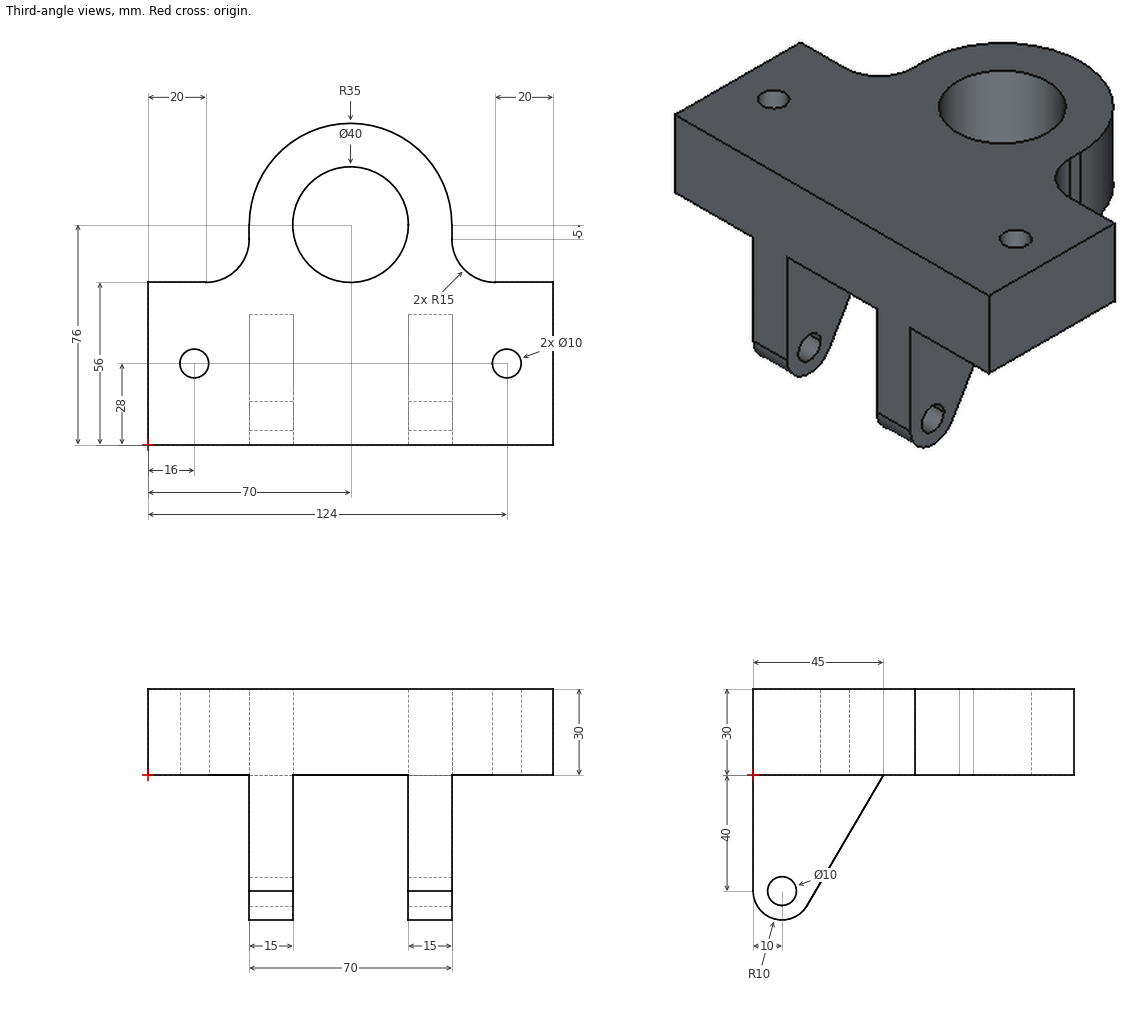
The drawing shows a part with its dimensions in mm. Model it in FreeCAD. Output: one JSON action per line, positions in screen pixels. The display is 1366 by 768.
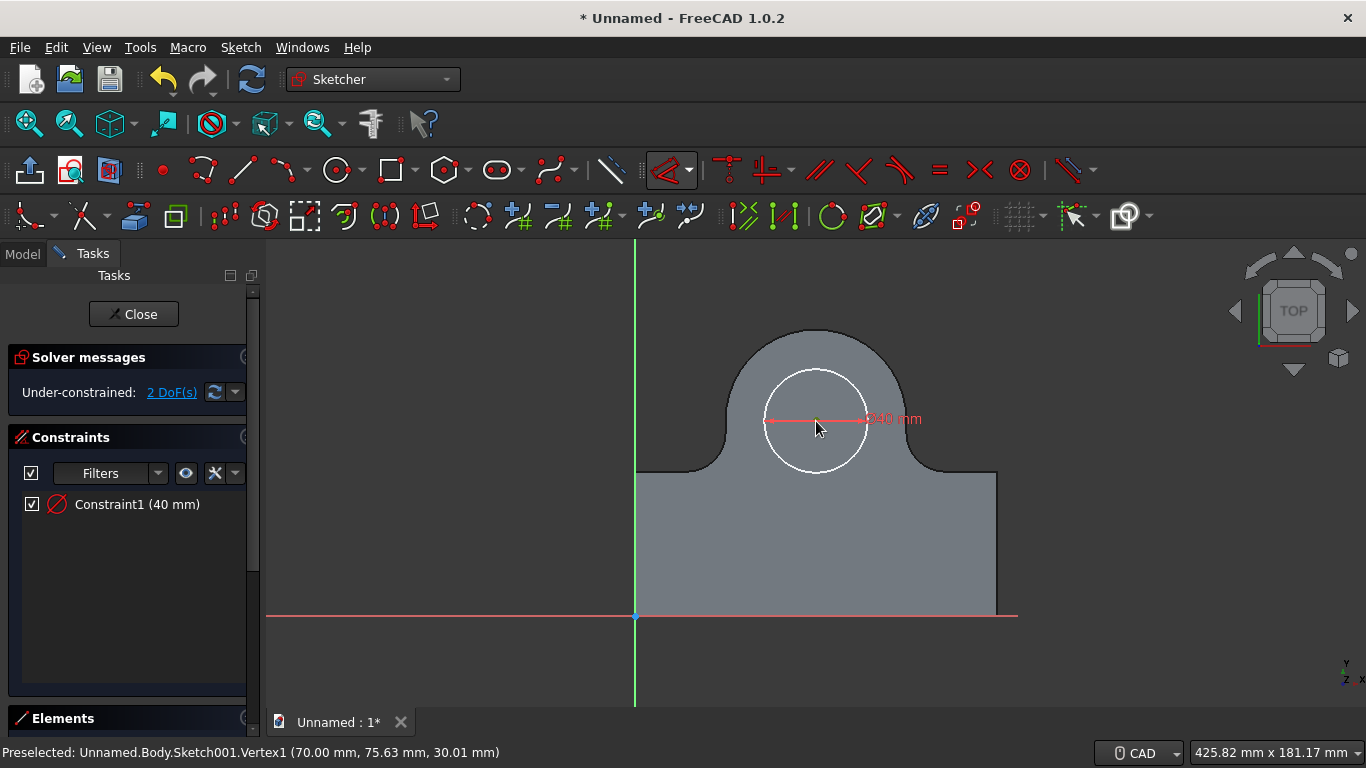
{"action": "left_click", "coordinate": [692, 170]}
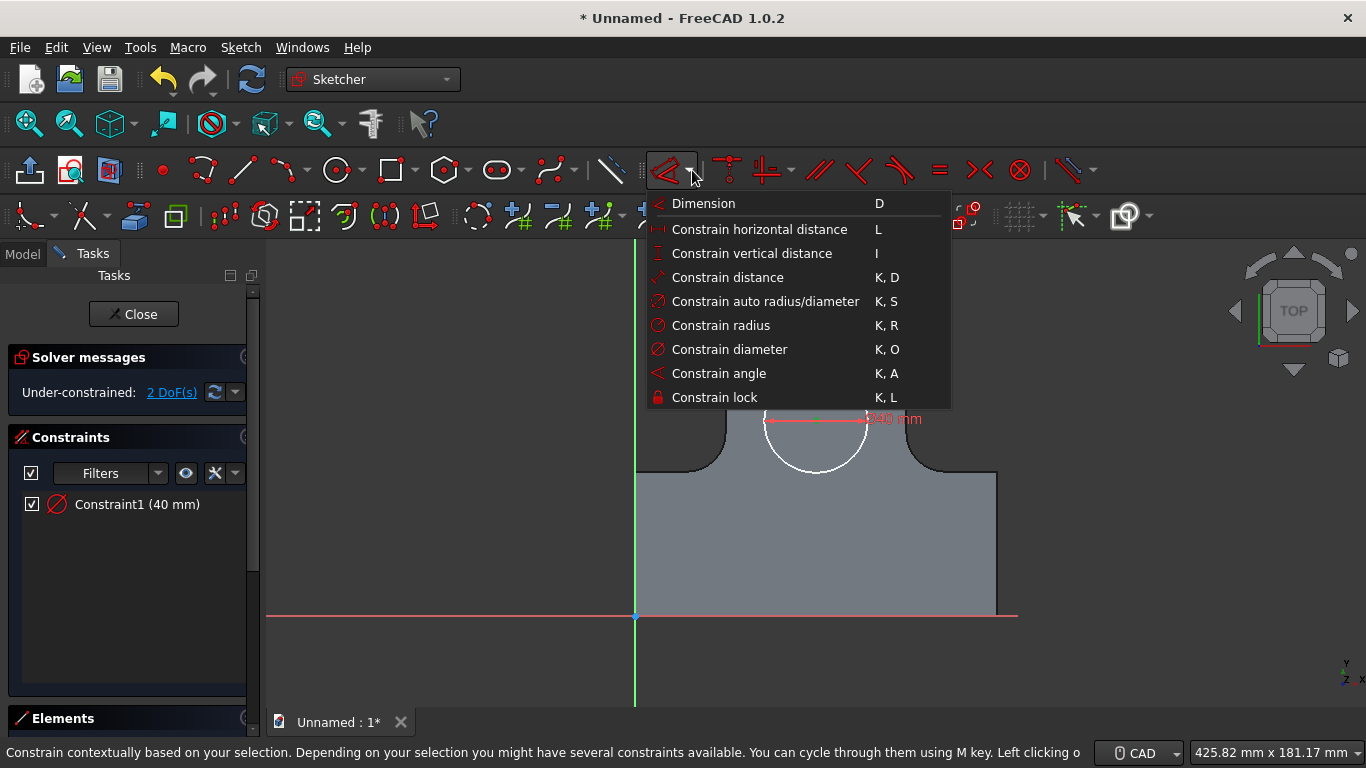
{"action": "left_click", "coordinate": [799, 229]}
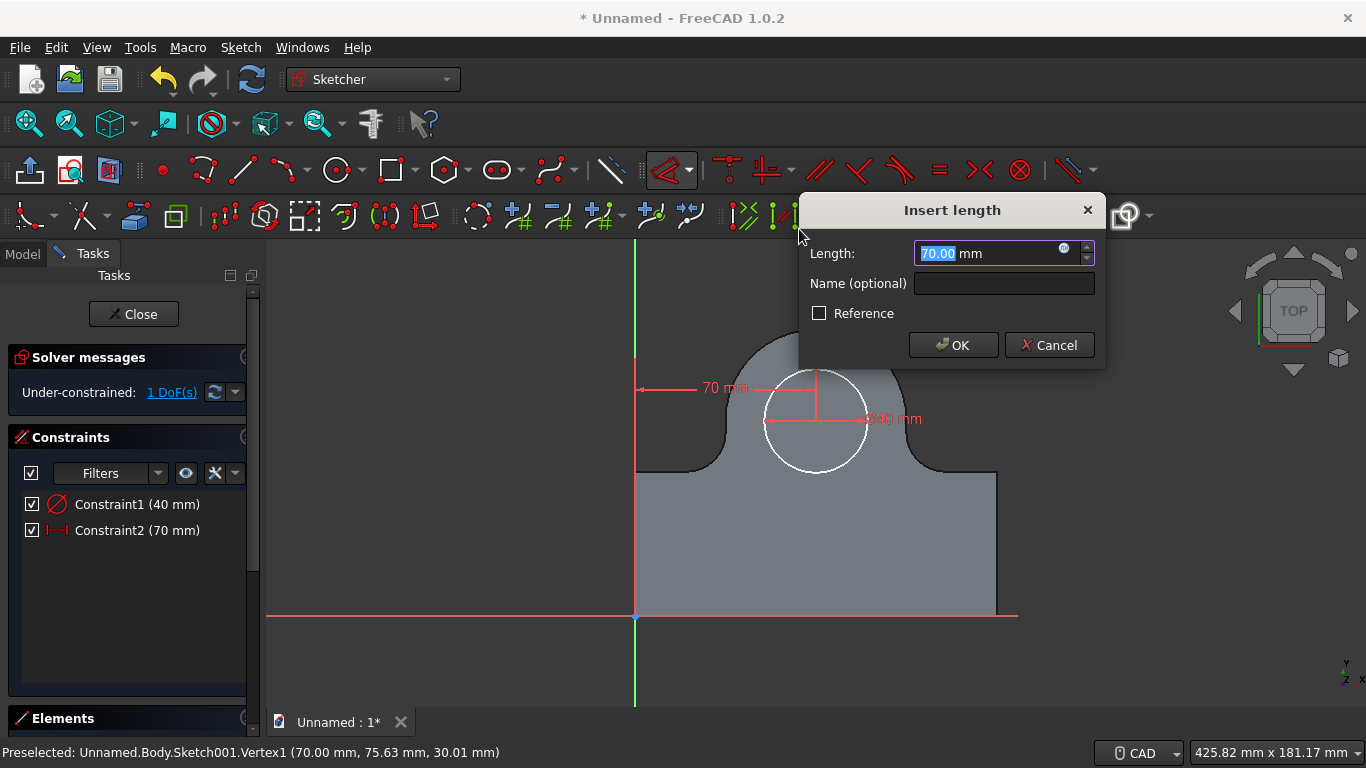
{"action": "type", "text": "70"}
{"action": "key", "text": "Return"}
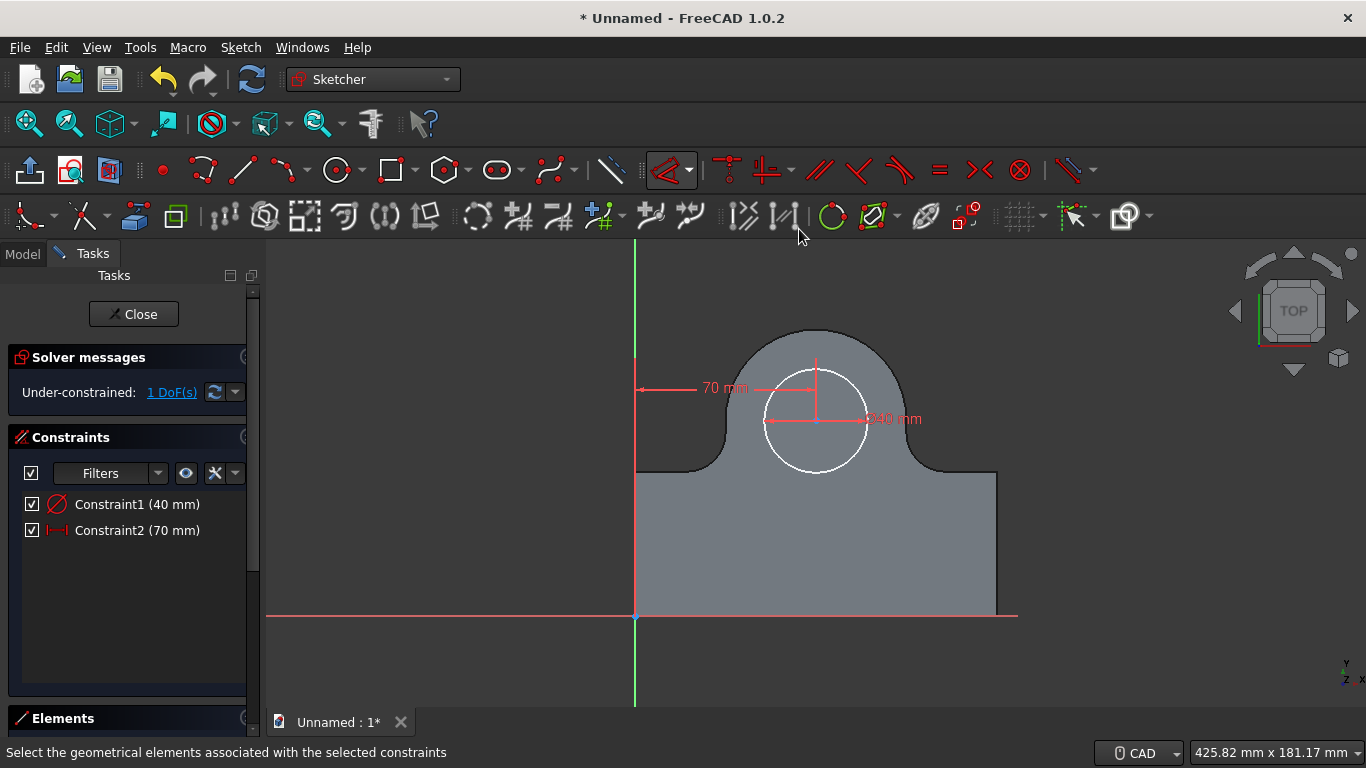
{"action": "left_click", "coordinate": [816, 421]}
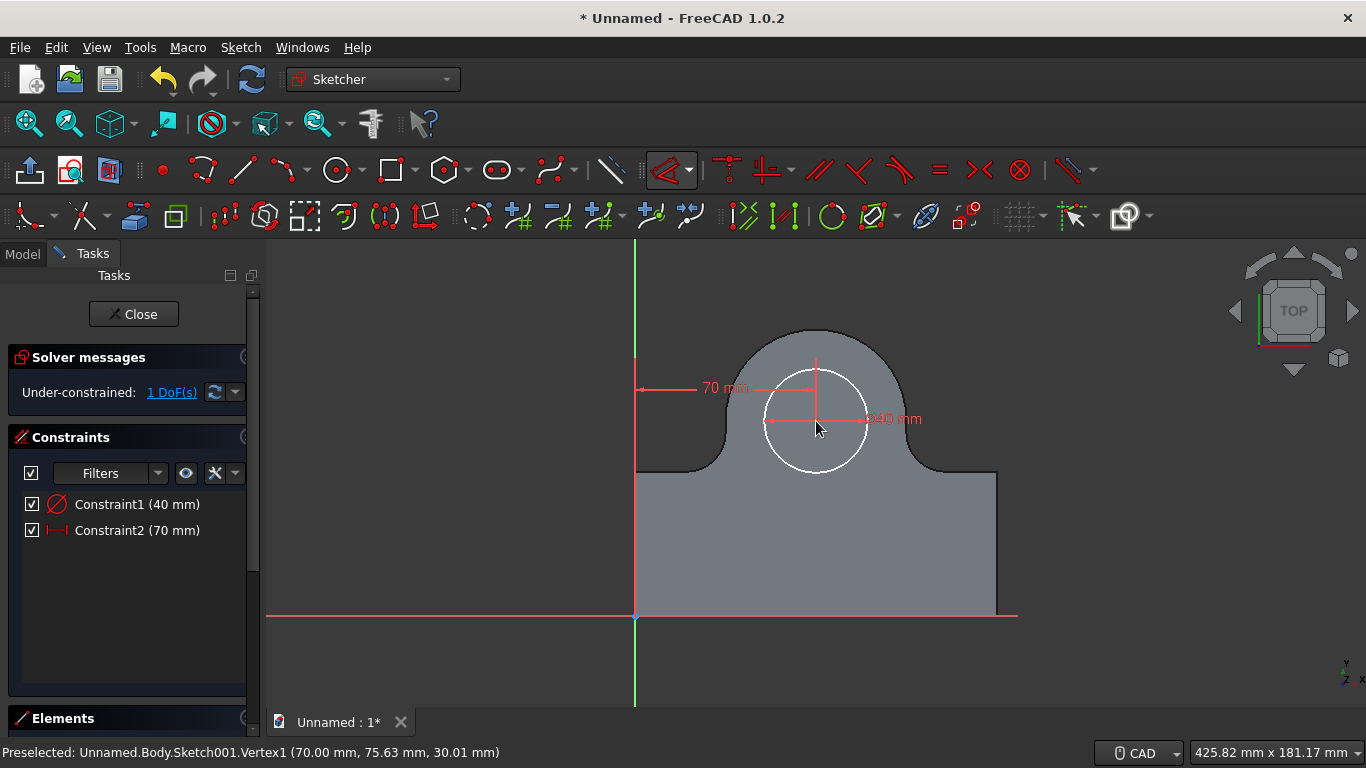
{"action": "key", "text": "i"}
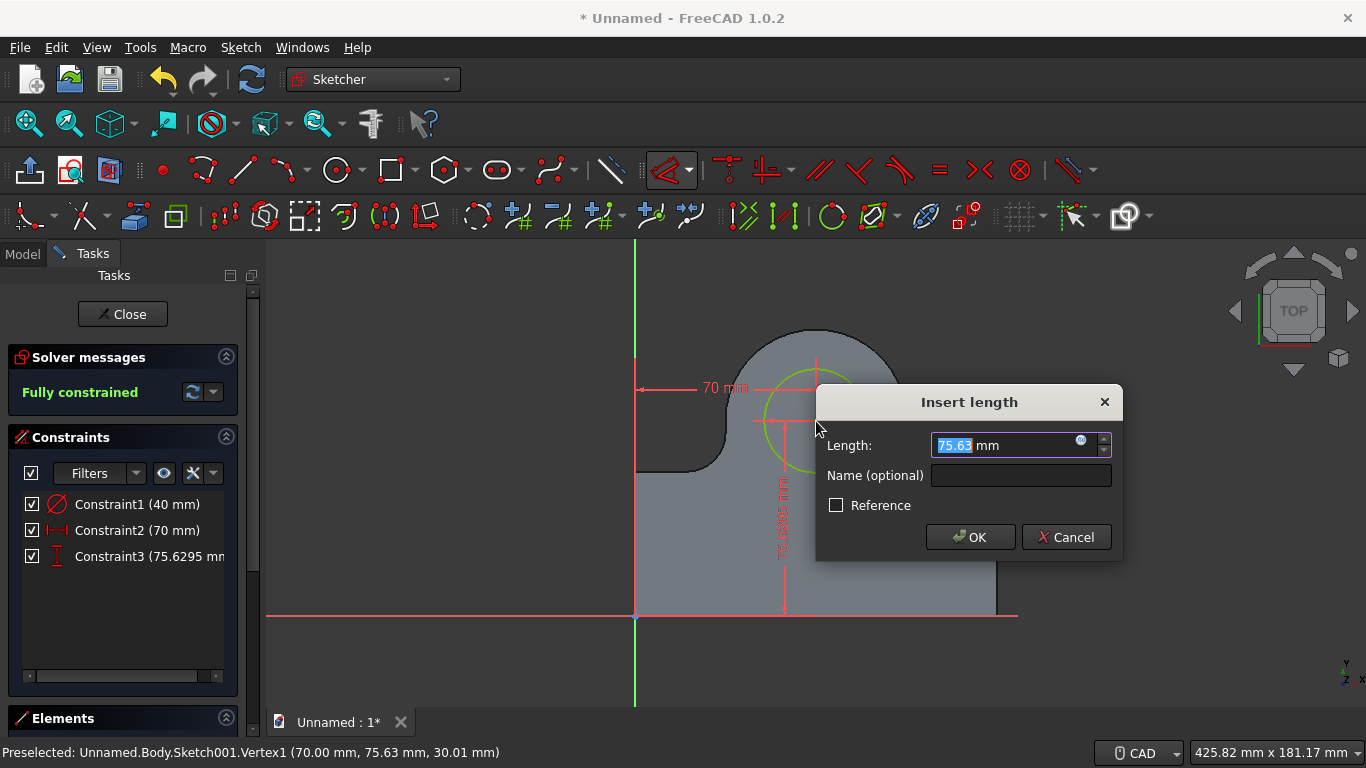
{"action": "type", "text": "76"}
{"action": "key", "text": "Return"}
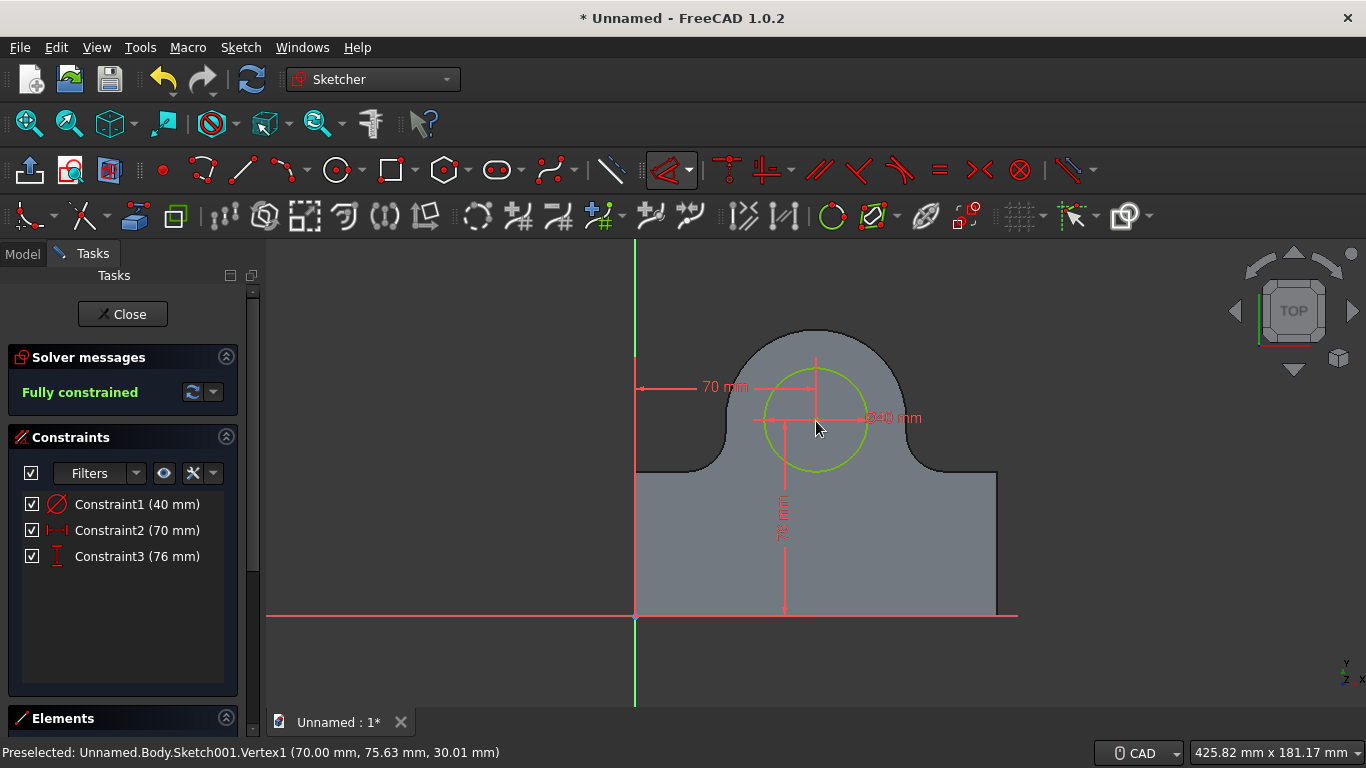
{"action": "left_click", "coordinate": [123, 314]}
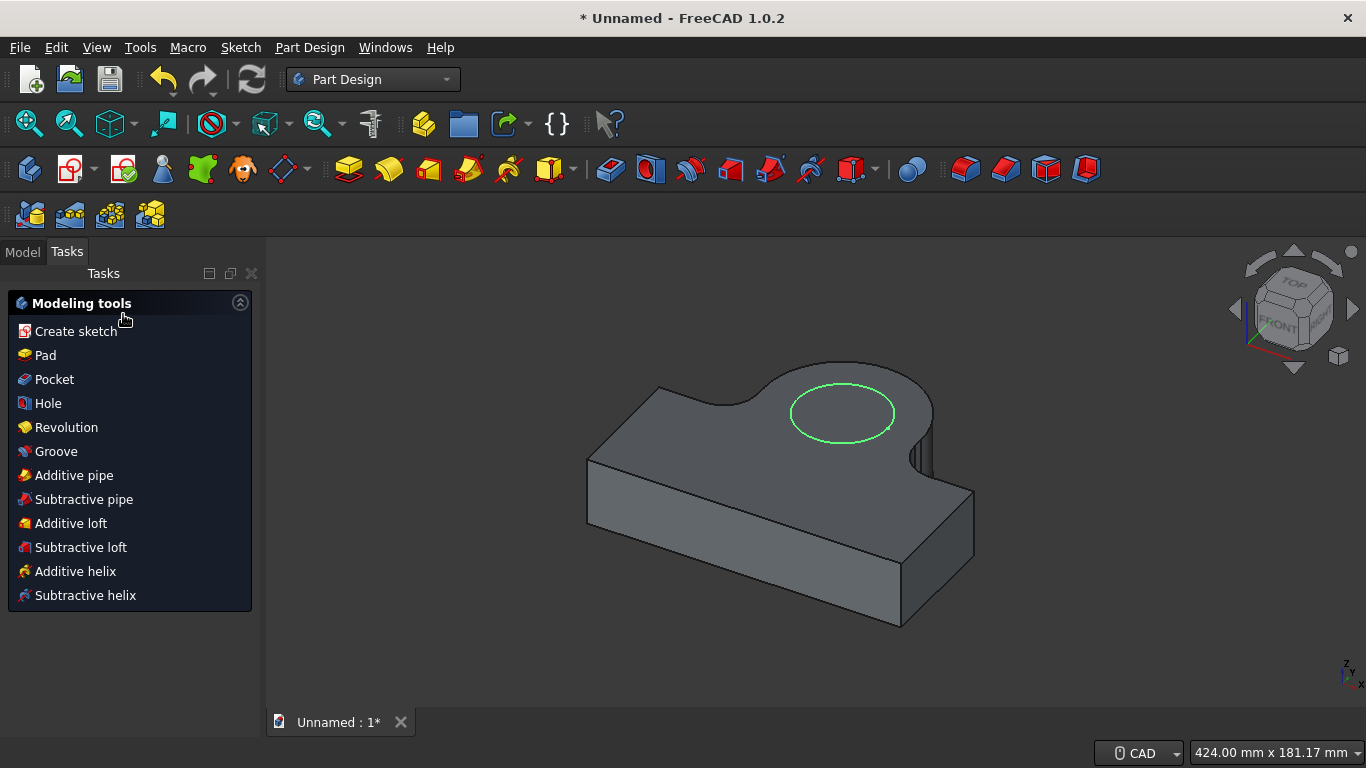
{"action": "left_click", "coordinate": [612, 170]}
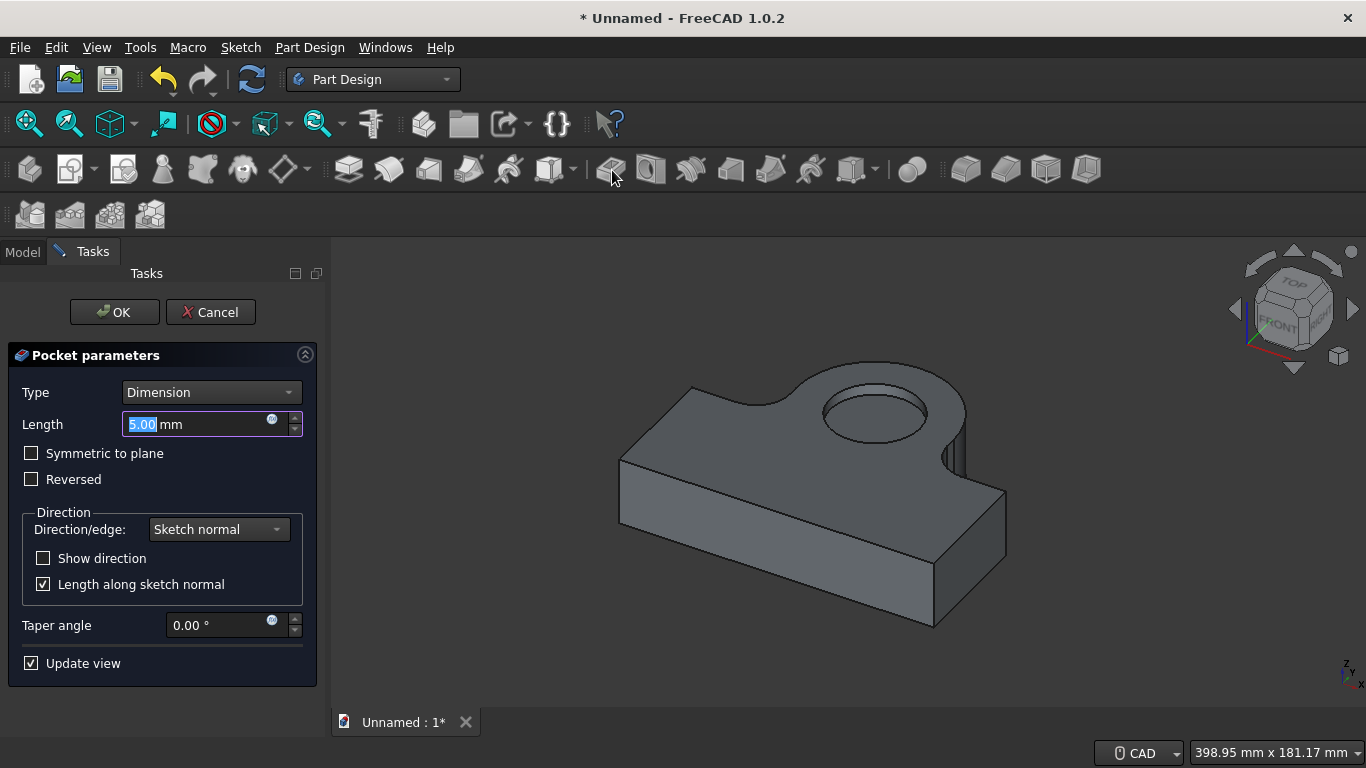
{"action": "type", "text": "30"}
{"action": "key", "text": "Tab"}